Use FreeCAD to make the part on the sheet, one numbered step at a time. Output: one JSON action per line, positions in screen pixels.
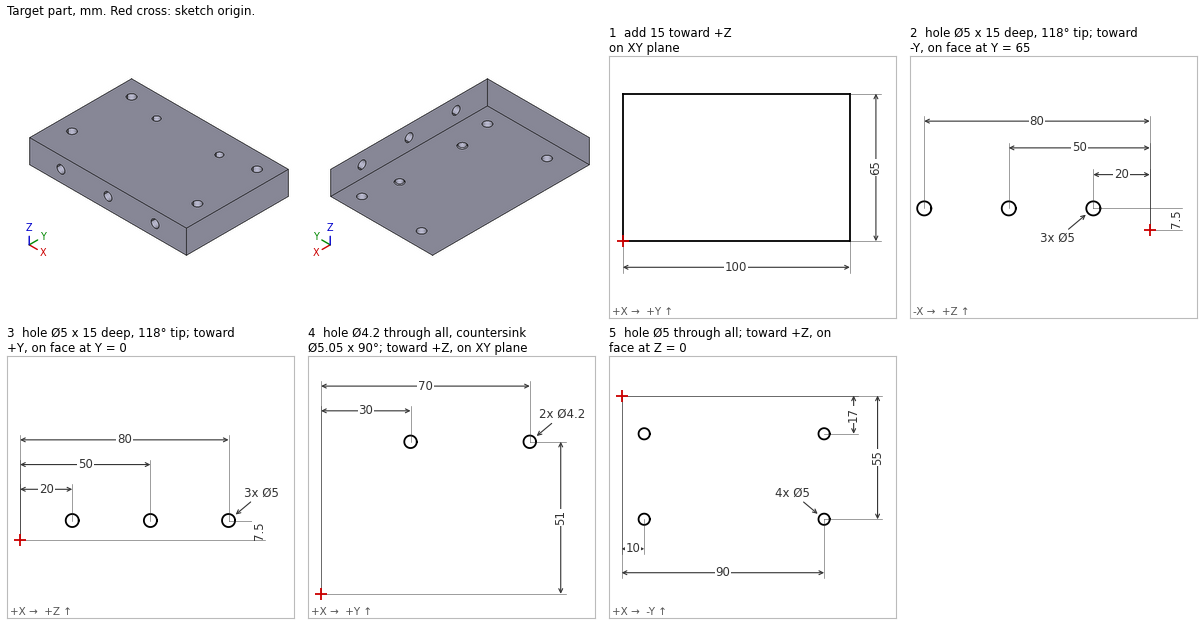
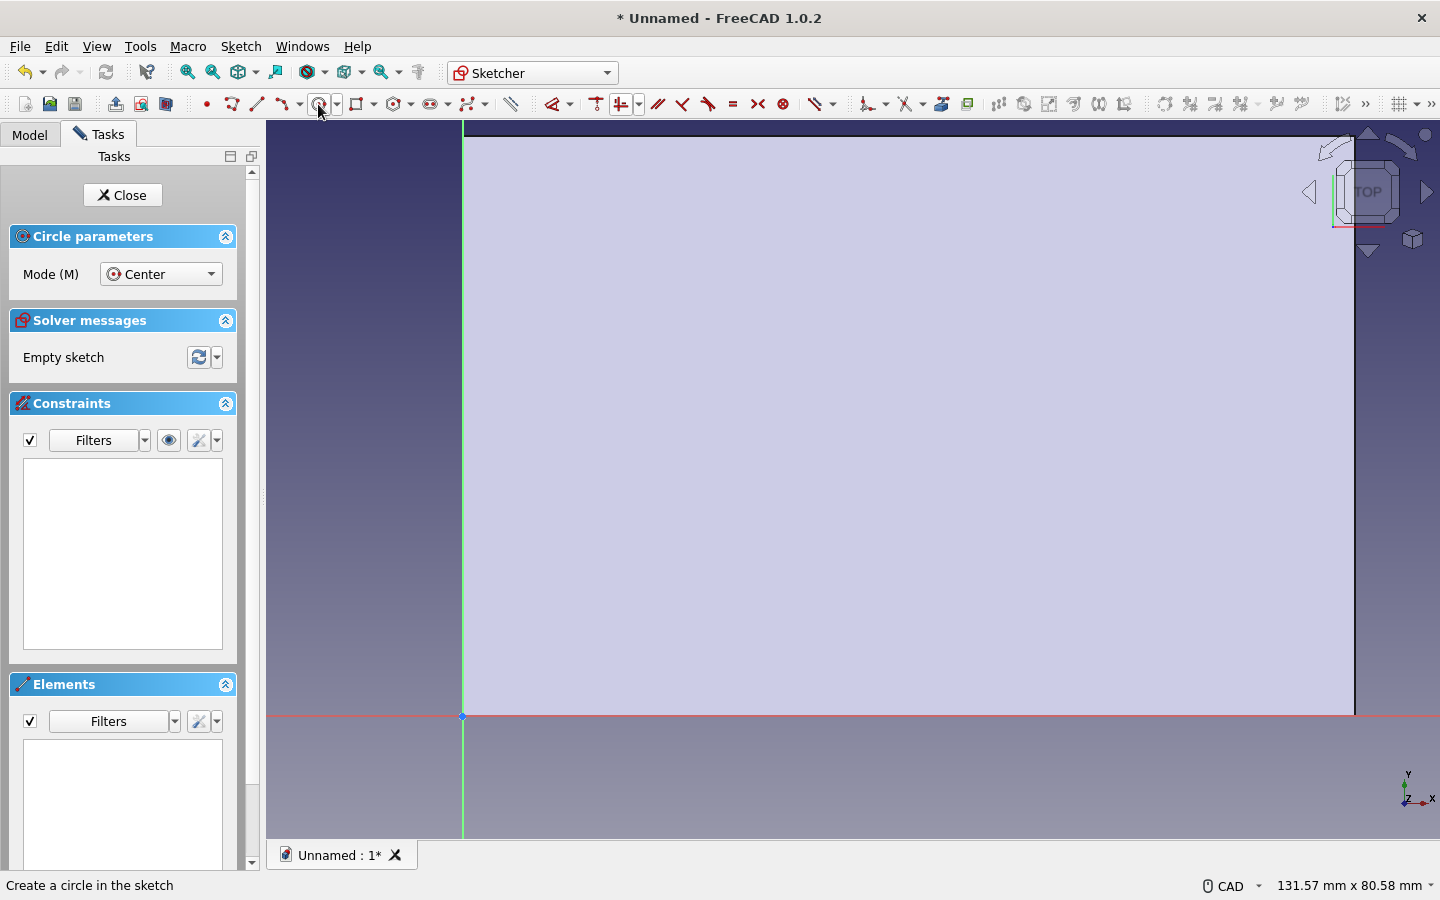
{"action": "left_click", "coordinate": [1087, 261]}
{"action": "mouse_move", "coordinate": [1101, 248]}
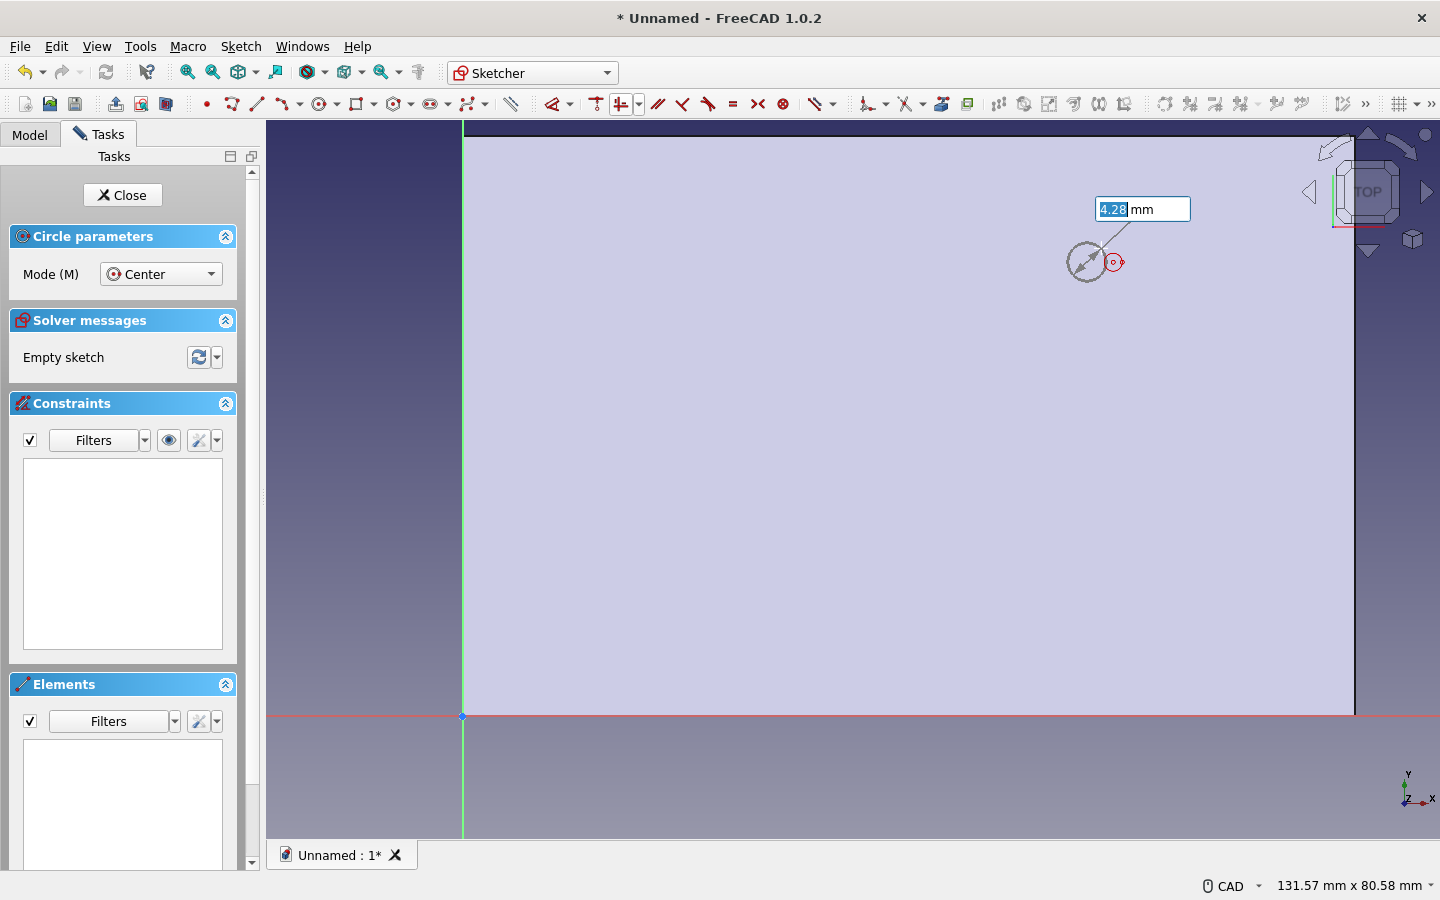
{"action": "type", "text": "4.2"}
{"action": "key", "text": "Return"}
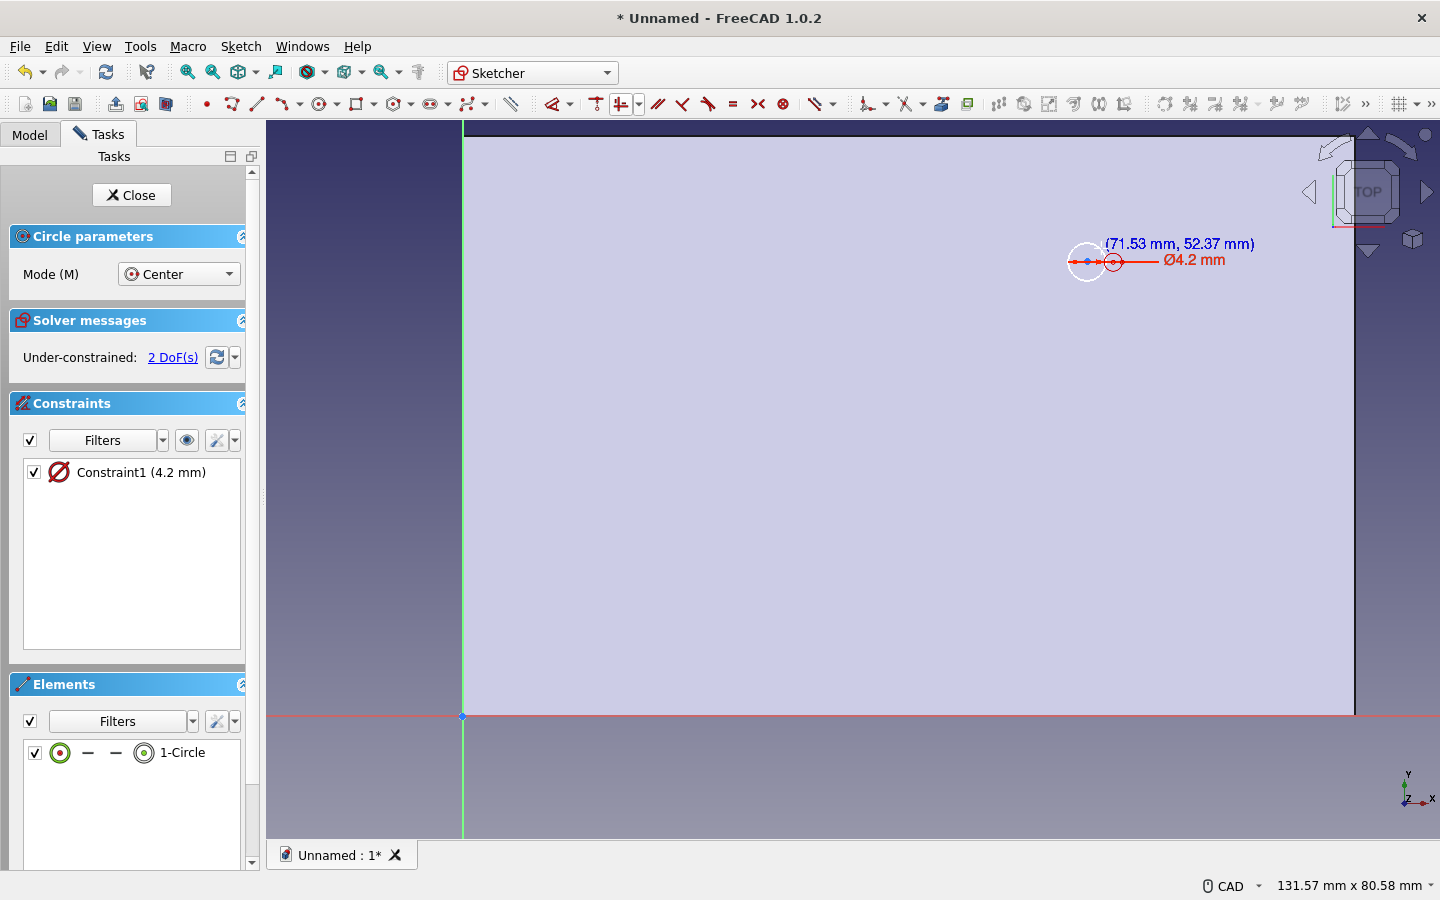
{"action": "left_click", "coordinate": [730, 261]}
{"action": "mouse_move", "coordinate": [744, 248]}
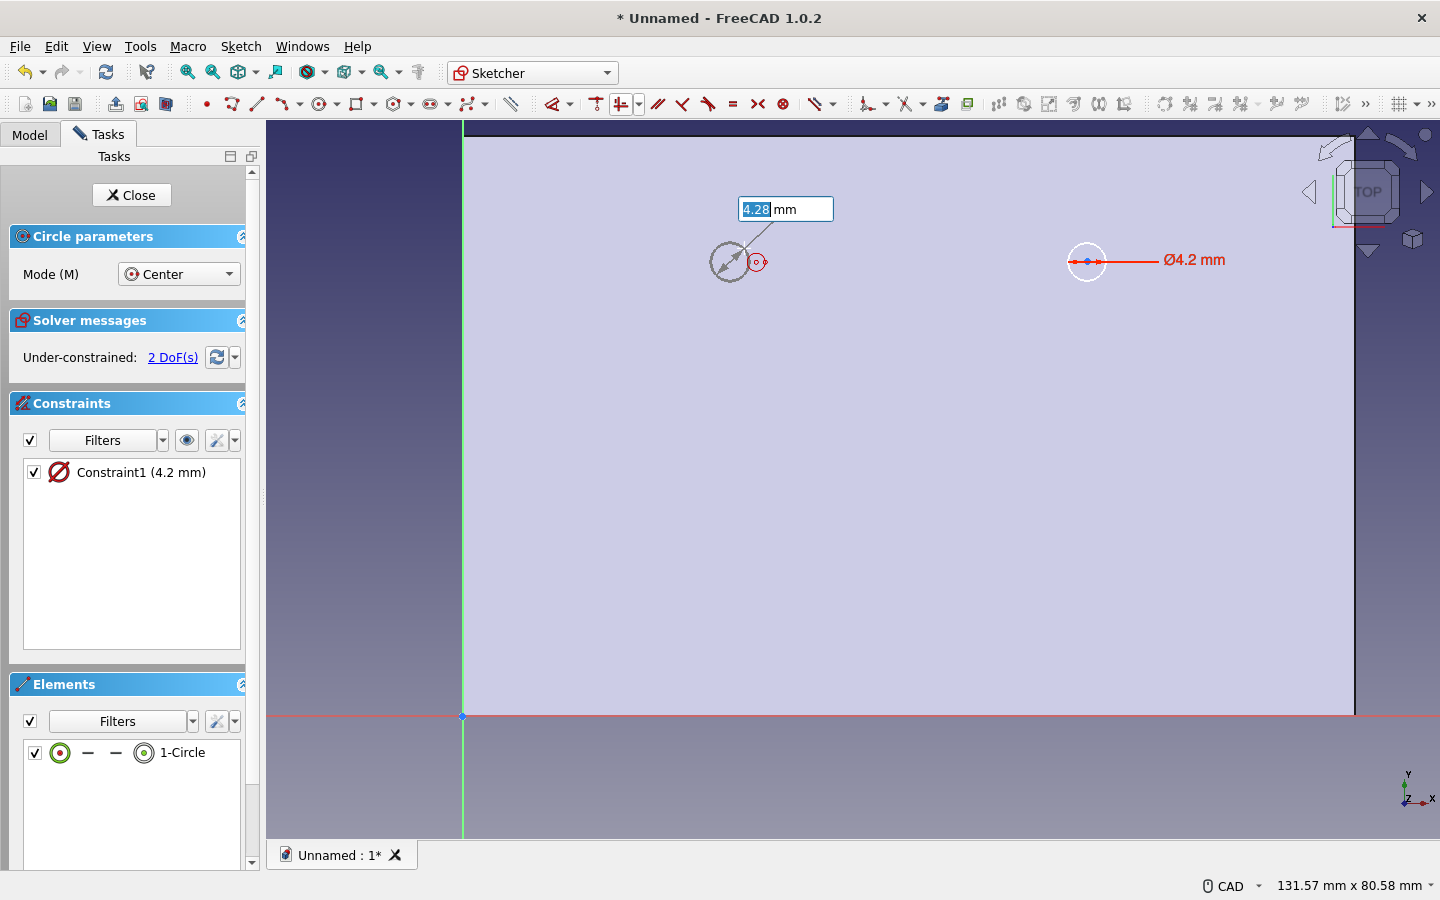
{"action": "type", "text": "4.2"}
{"action": "key", "text": "Return"}
{"action": "key", "text": "Escape"}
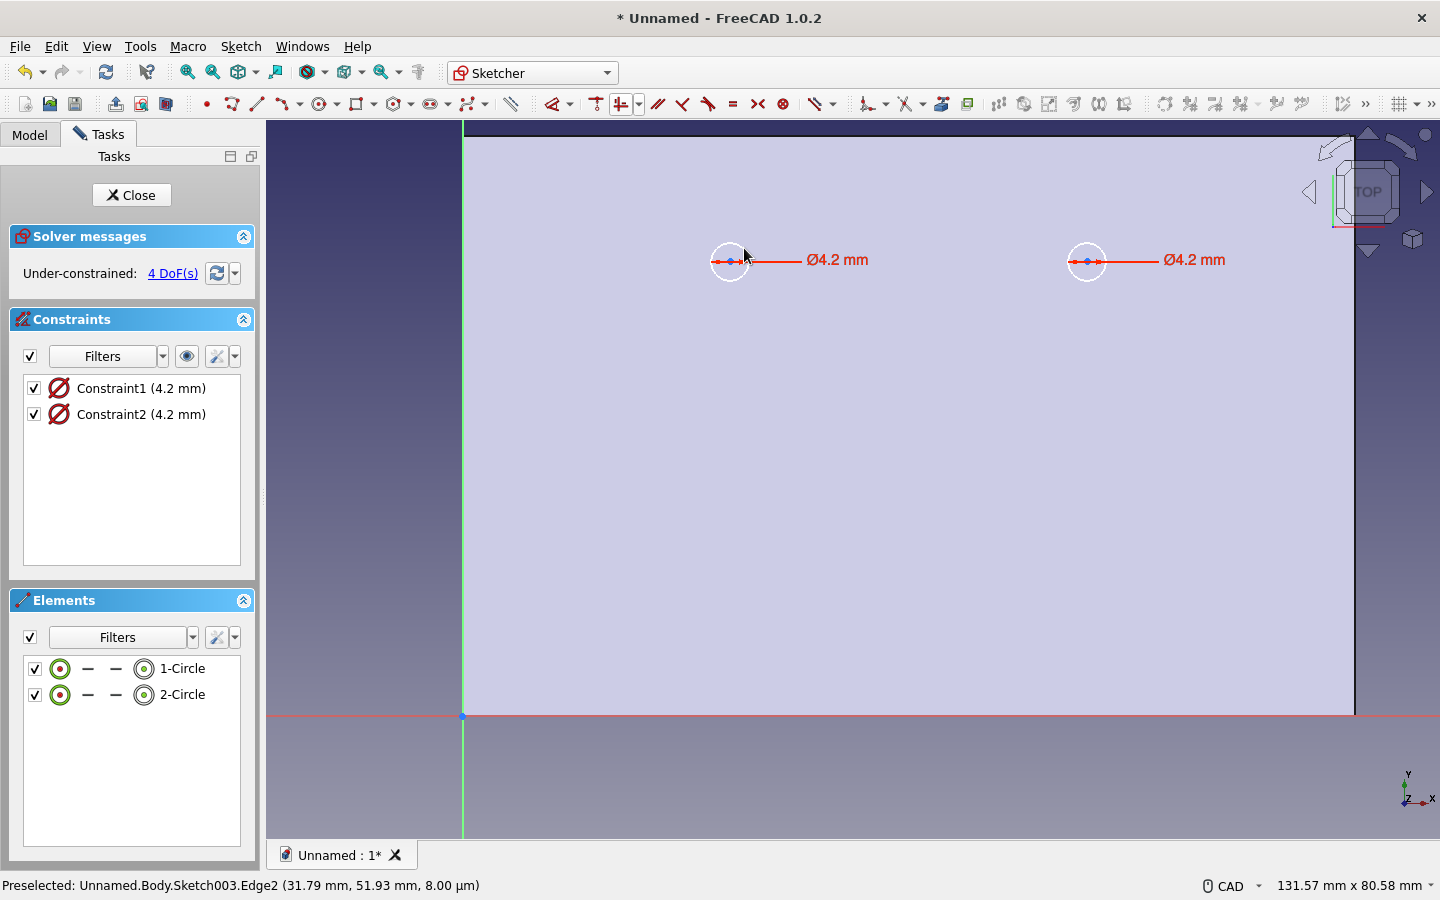
{"action": "left_click", "coordinate": [1087, 262]}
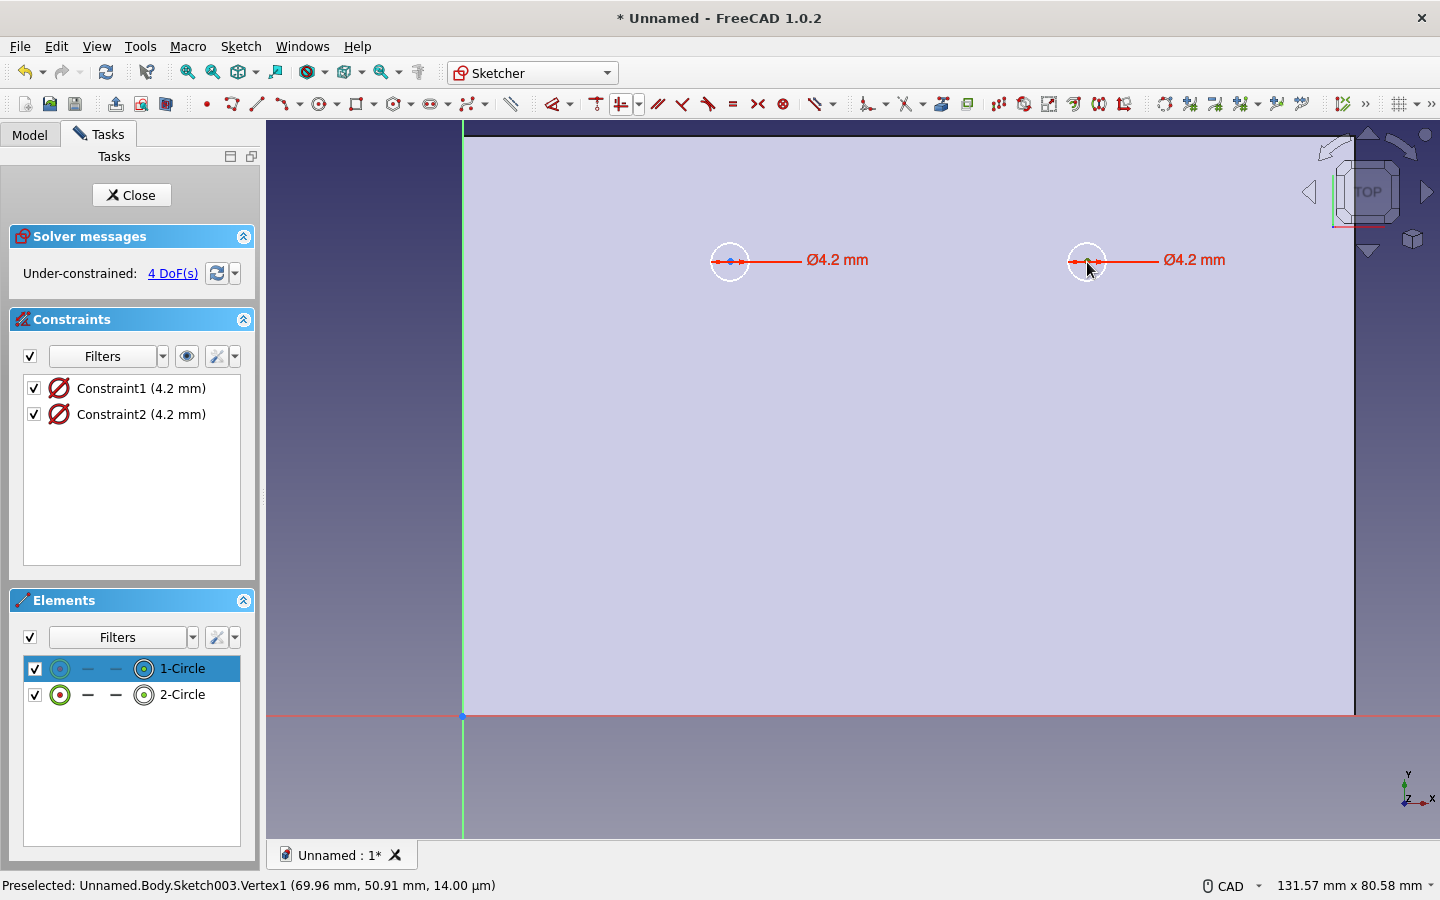
{"action": "left_click", "coordinate": [730, 262]}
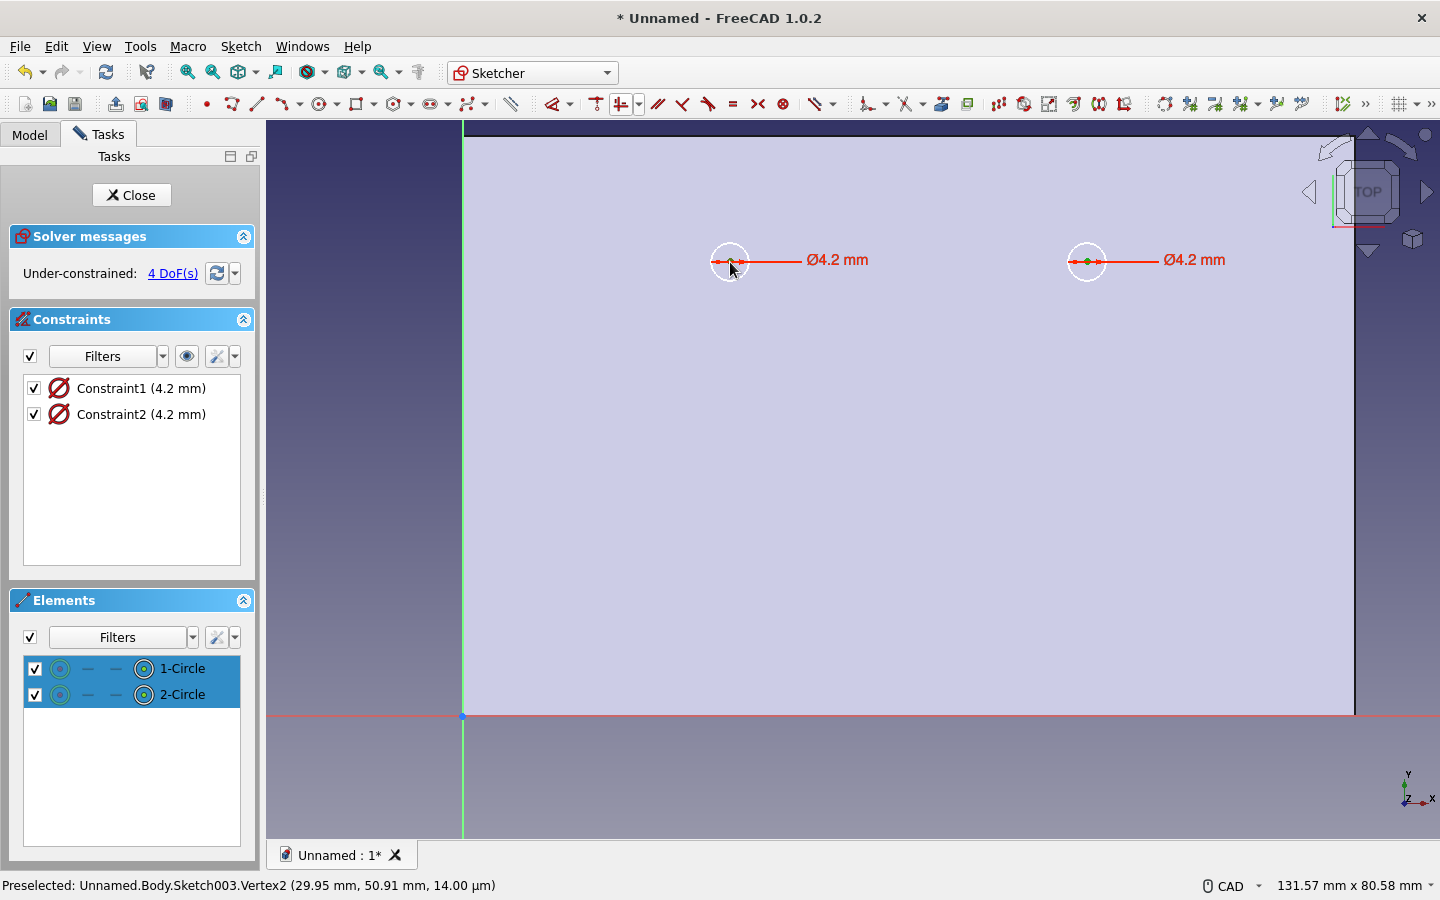
{"action": "left_click", "coordinate": [638, 104]}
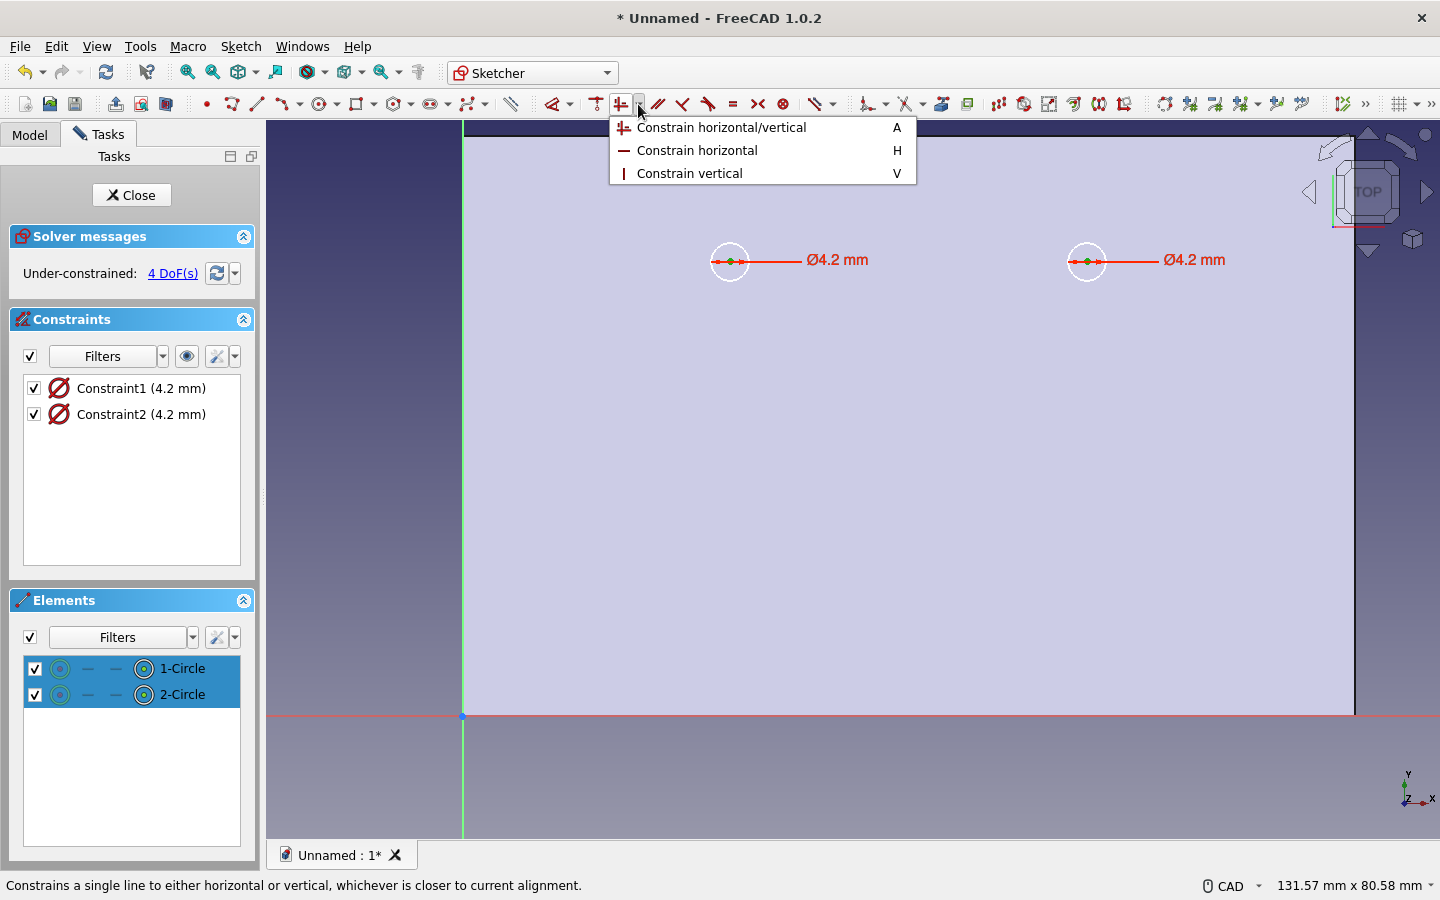
{"action": "left_click", "coordinate": [763, 150]}